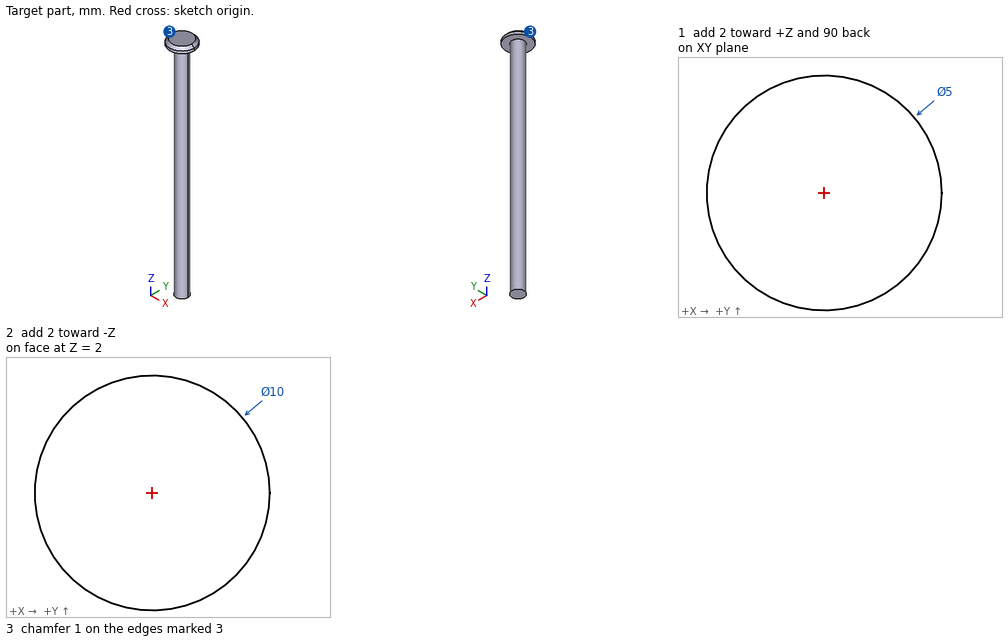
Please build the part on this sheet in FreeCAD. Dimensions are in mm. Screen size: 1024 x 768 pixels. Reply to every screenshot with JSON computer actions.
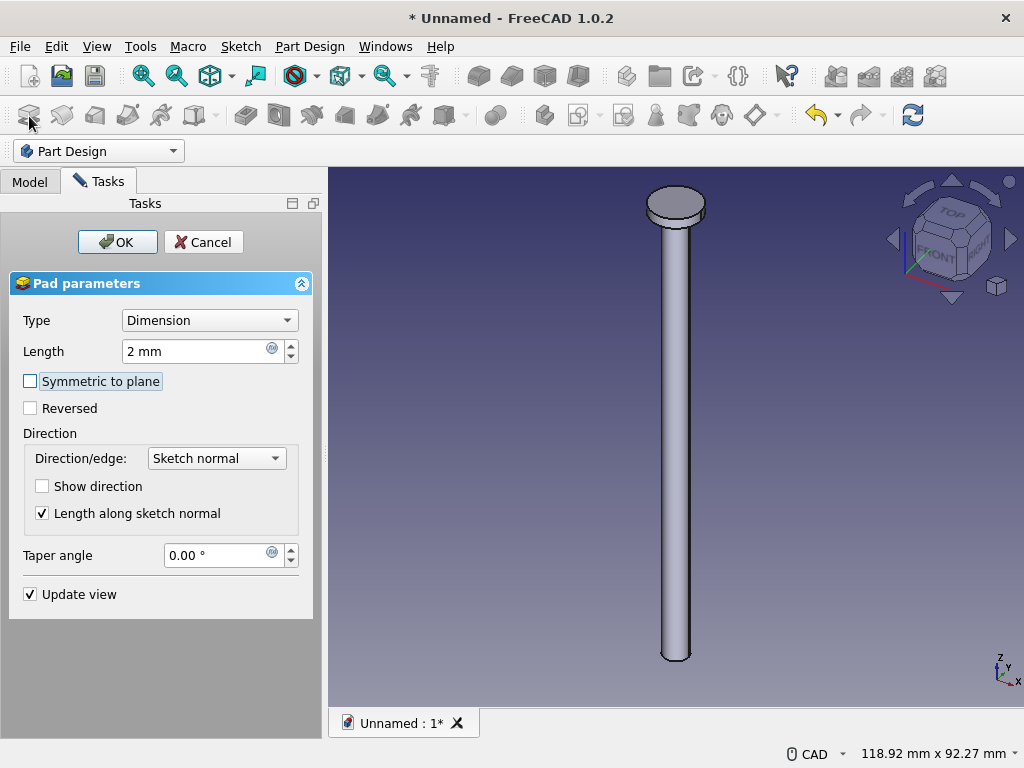
{"action": "left_click", "coordinate": [31, 408]}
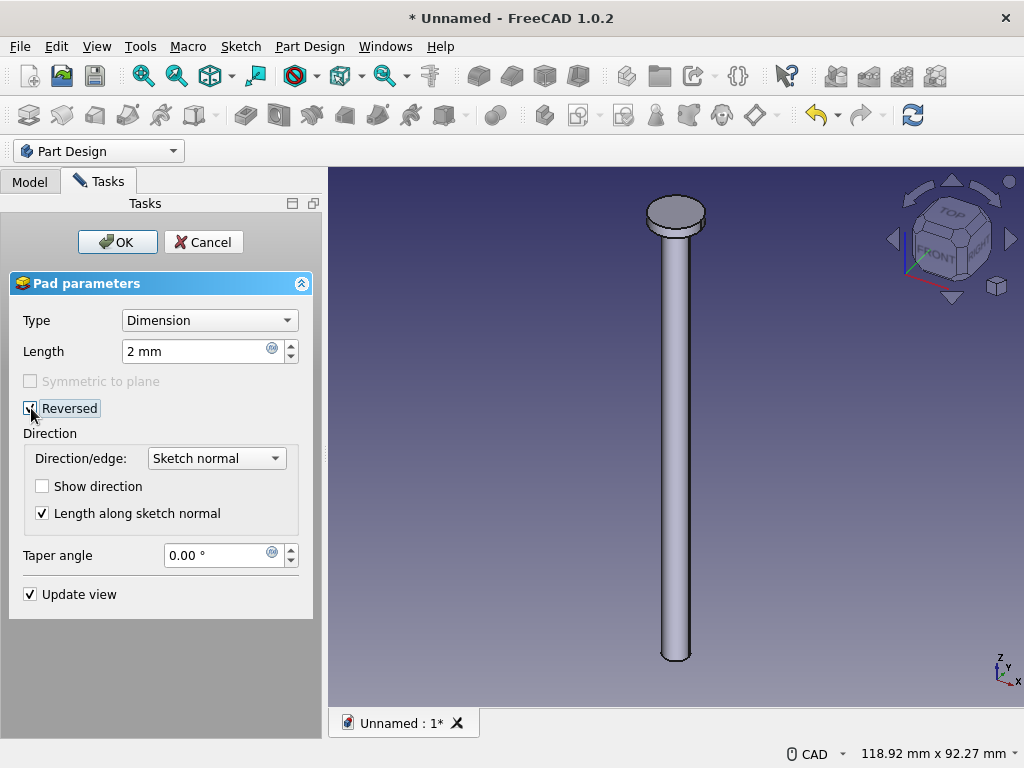
{"action": "left_click", "coordinate": [118, 242]}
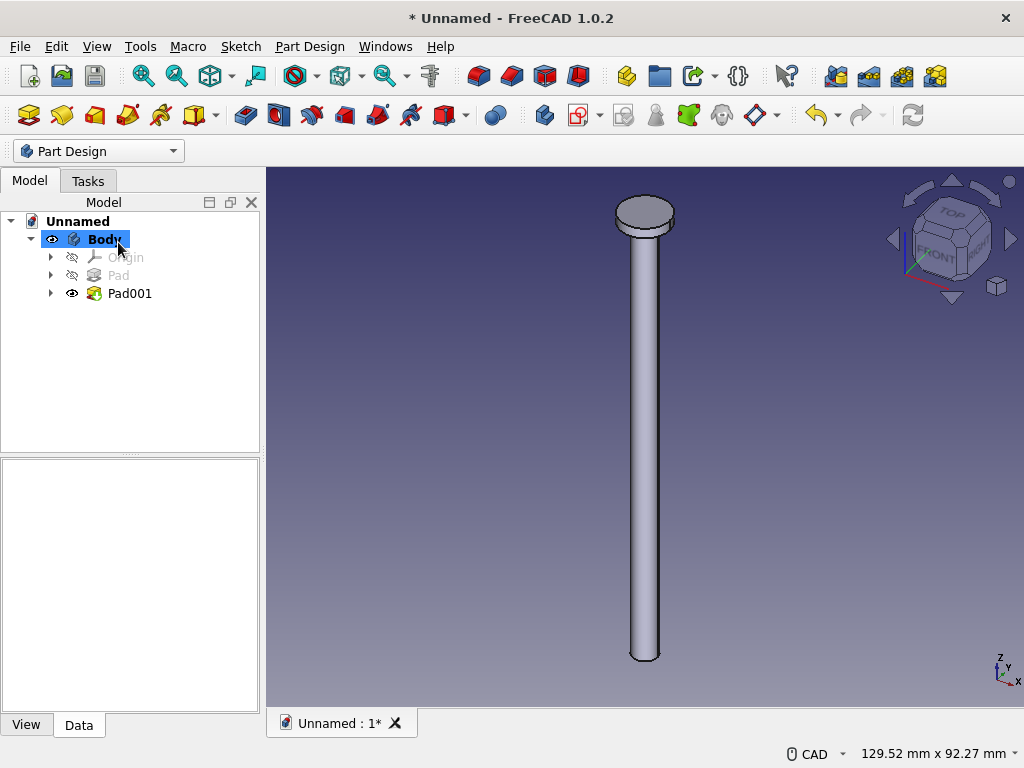
{"action": "left_click", "coordinate": [616, 213]}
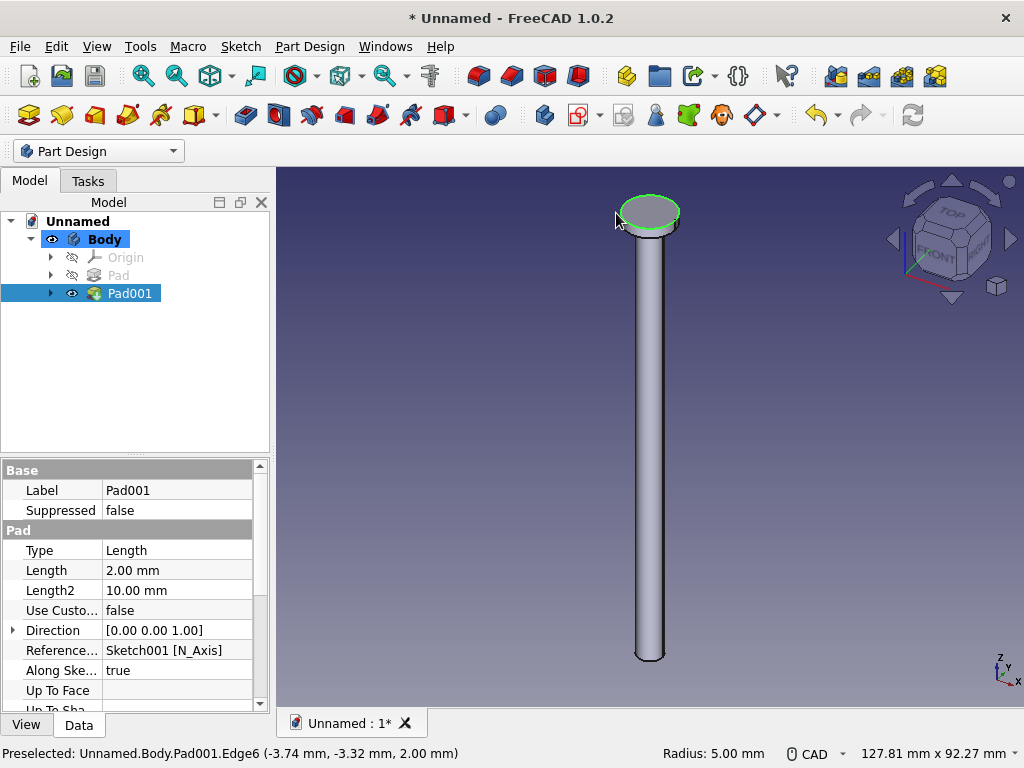
{"action": "left_click", "coordinate": [512, 76]}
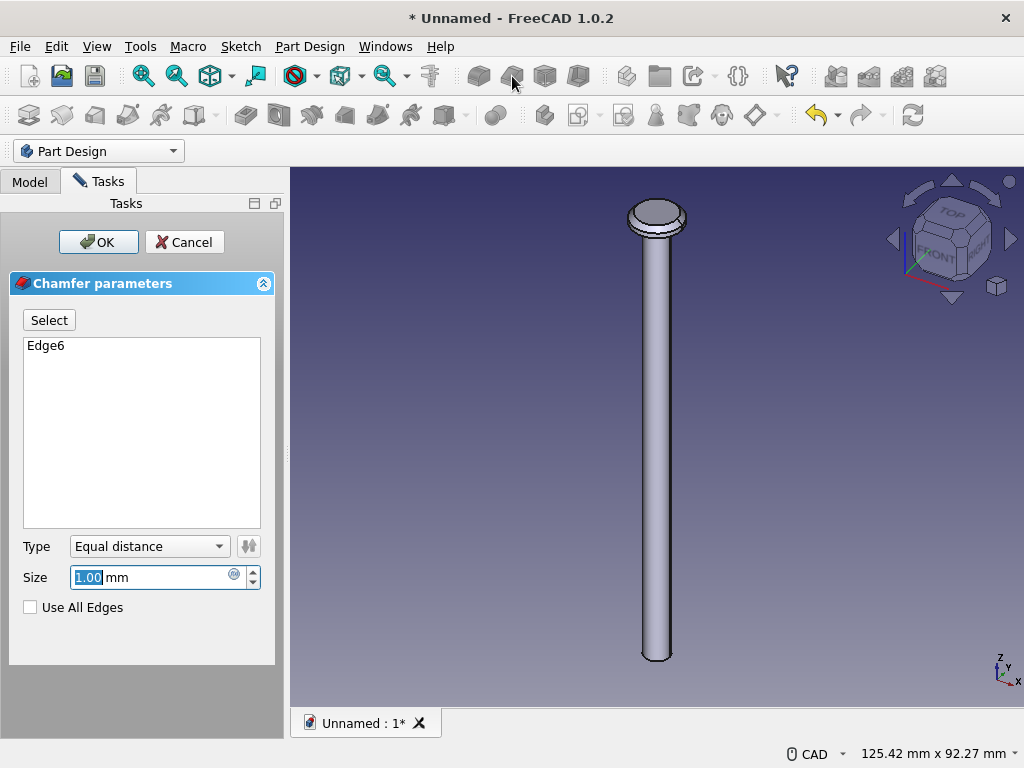
{"action": "type", "text": "1"}
{"action": "key", "text": "Tab"}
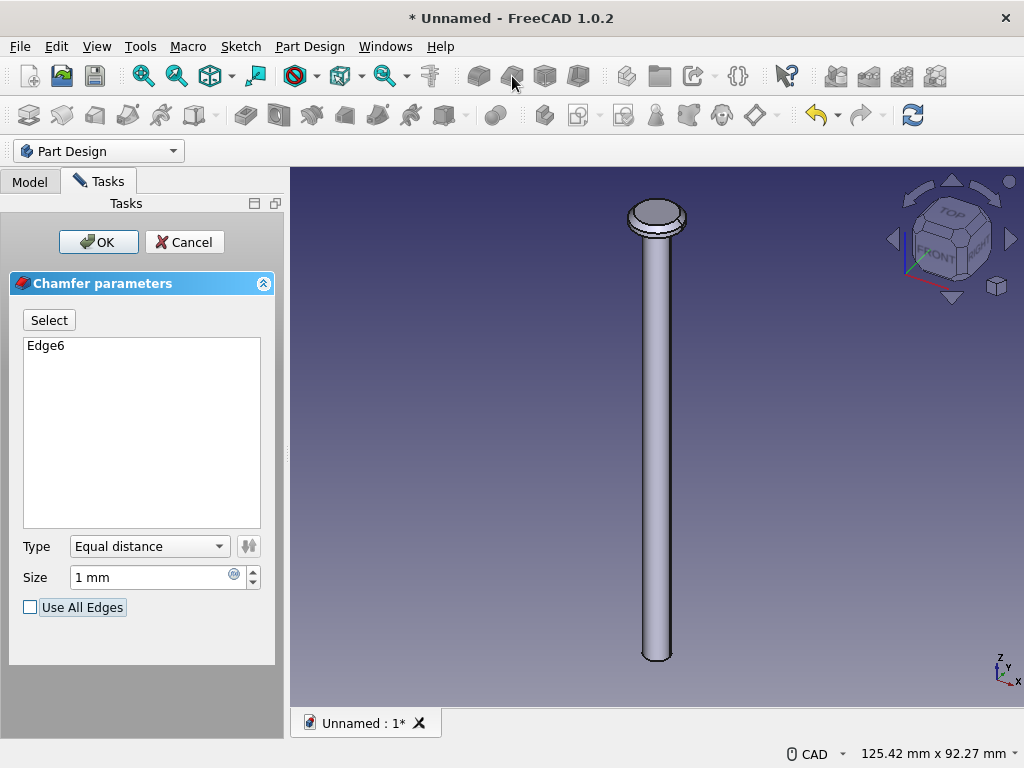
{"action": "left_click", "coordinate": [99, 242]}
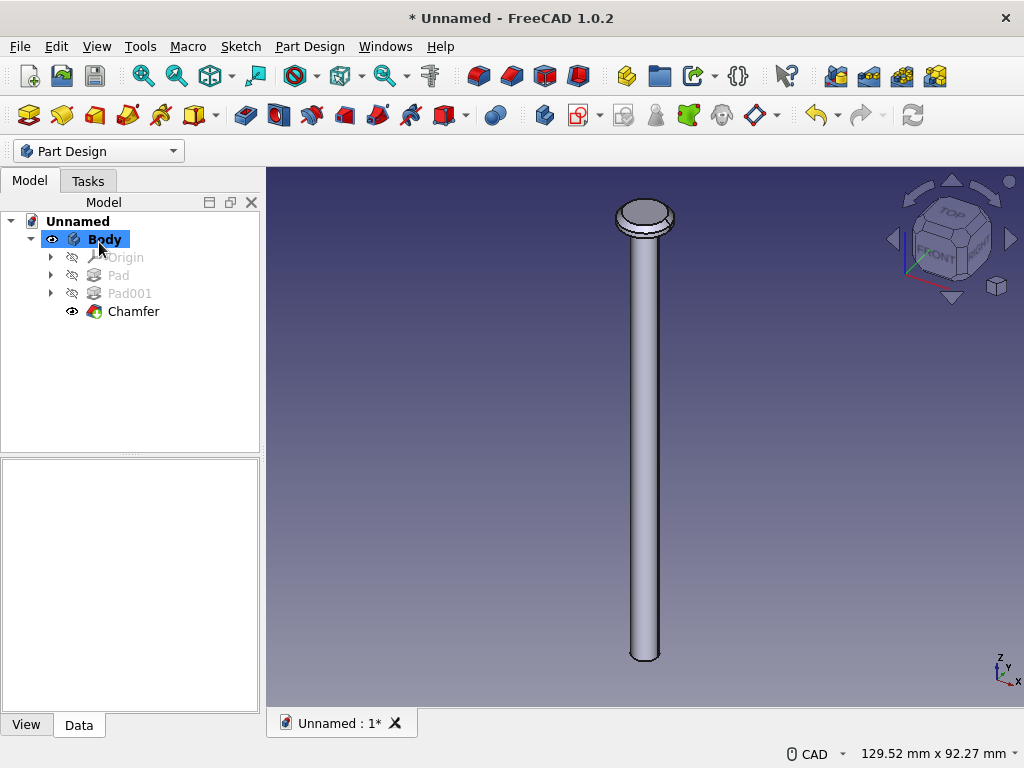
{"action": "key", "text": "0"}